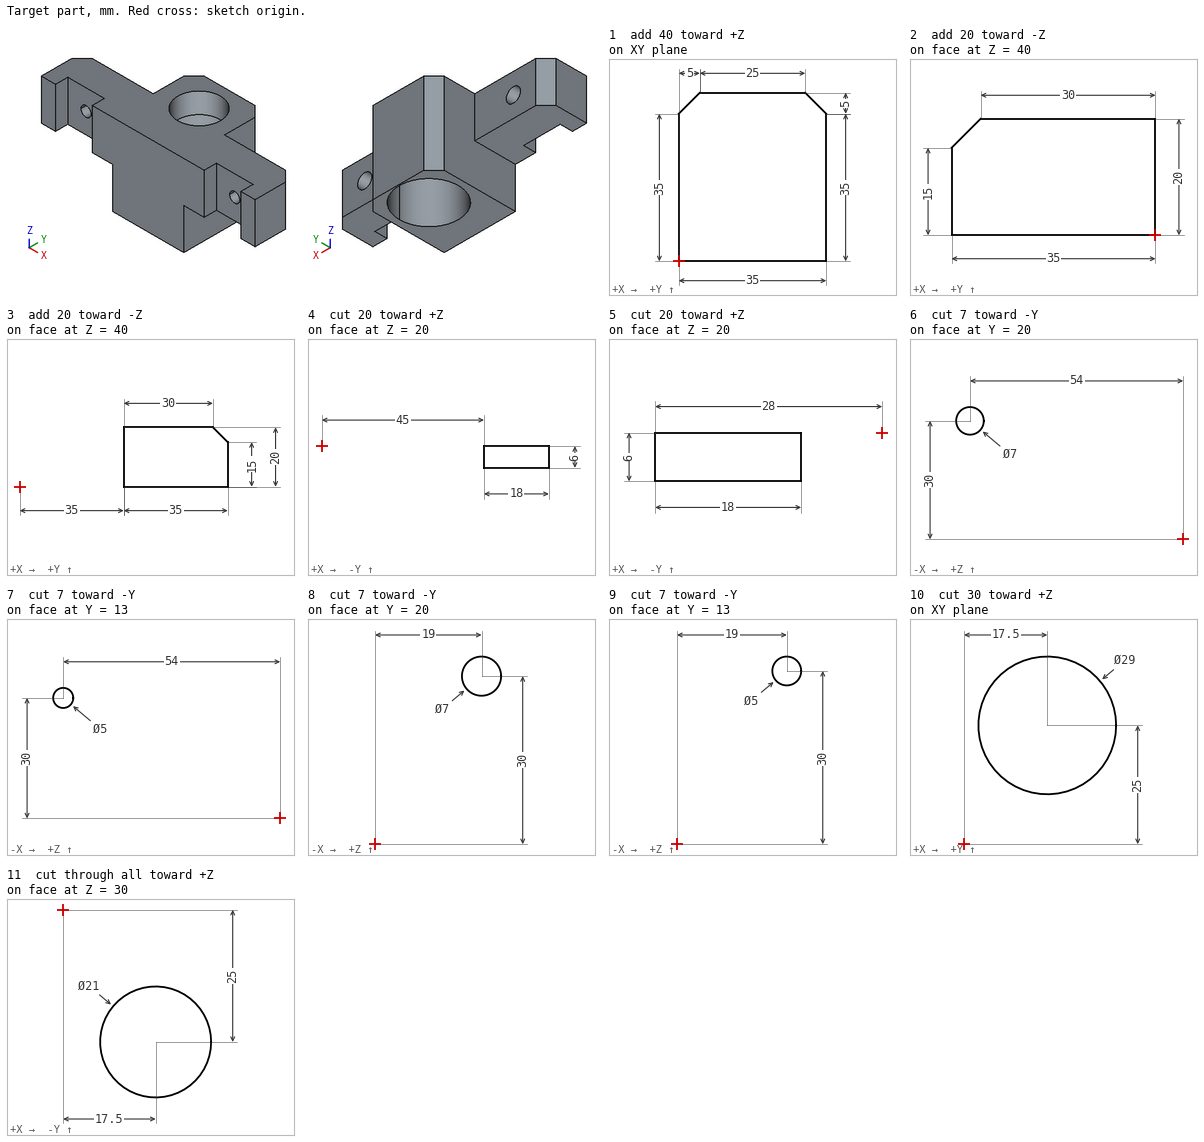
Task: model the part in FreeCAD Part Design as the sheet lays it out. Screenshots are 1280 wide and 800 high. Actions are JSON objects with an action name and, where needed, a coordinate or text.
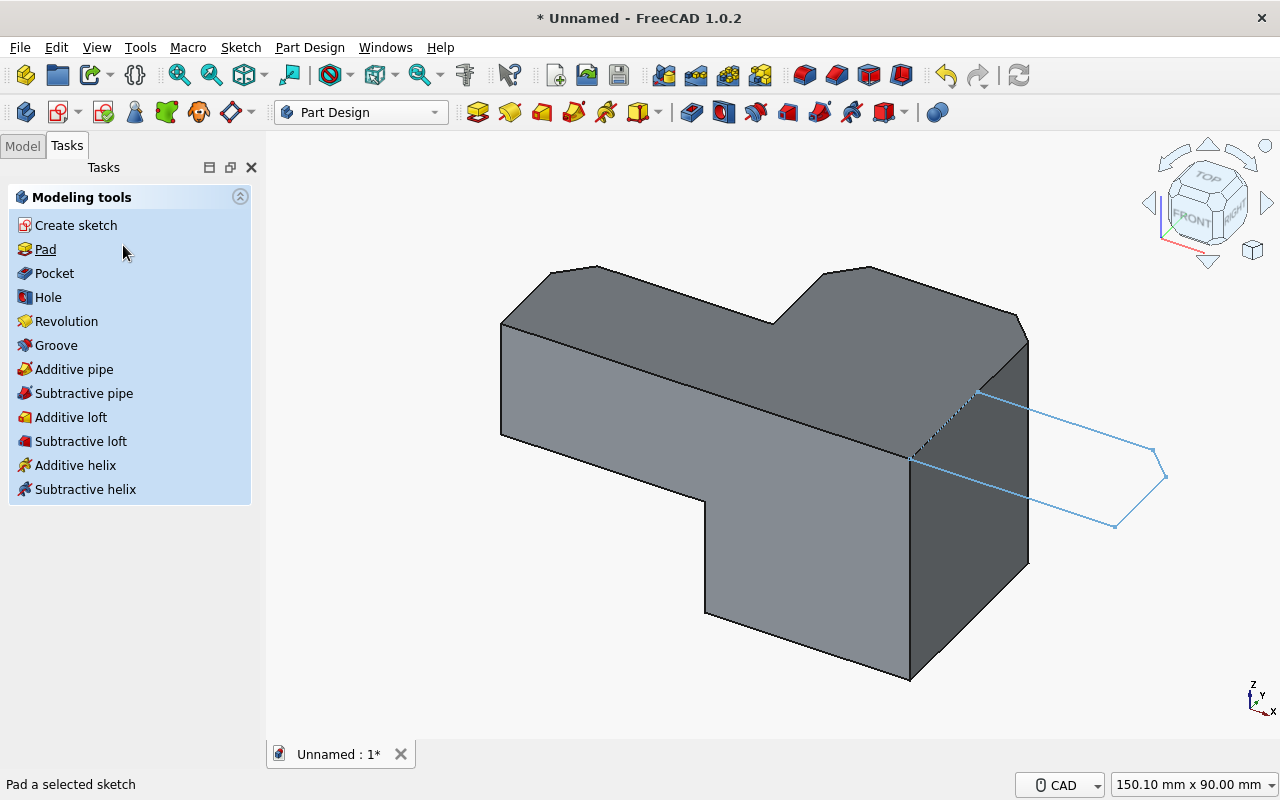
{"action": "left_click", "coordinate": [478, 112]}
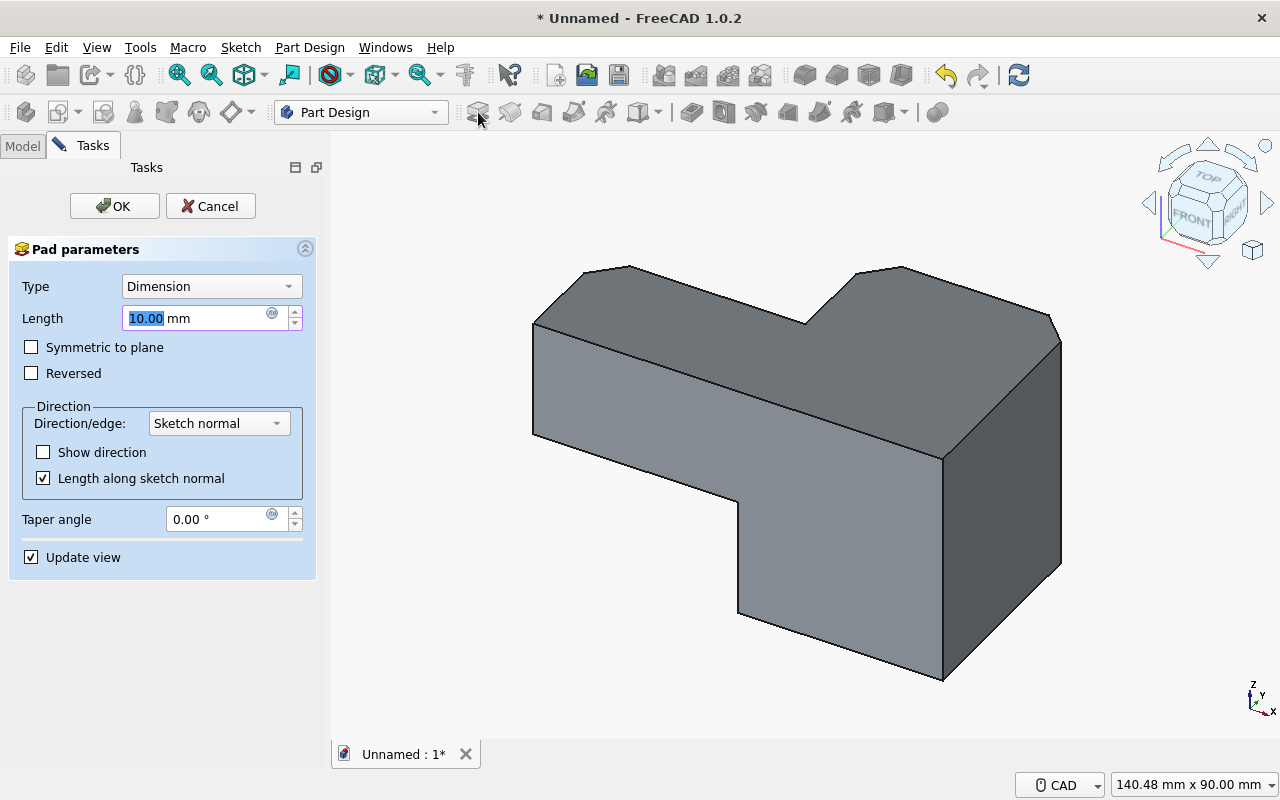
{"action": "type", "text": "20"}
{"action": "key", "text": "Tab"}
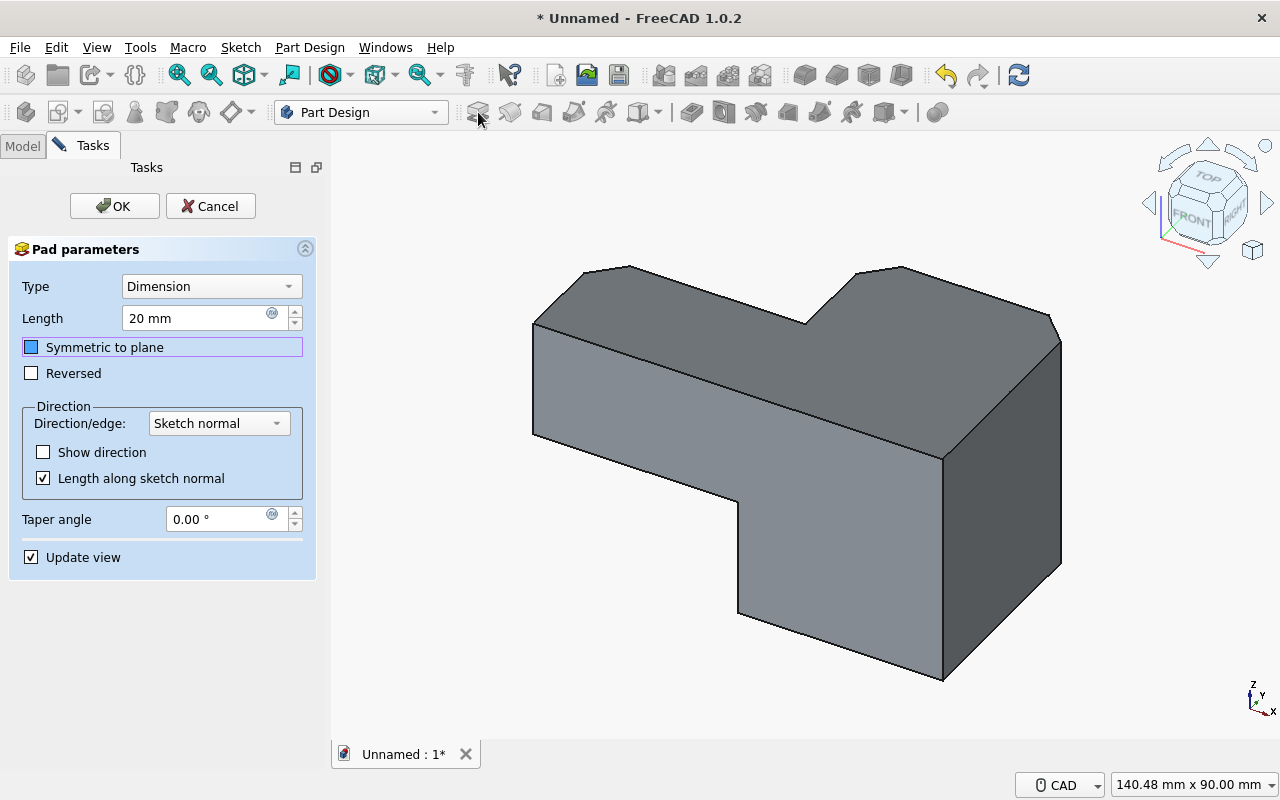
{"action": "left_click", "coordinate": [30, 373]}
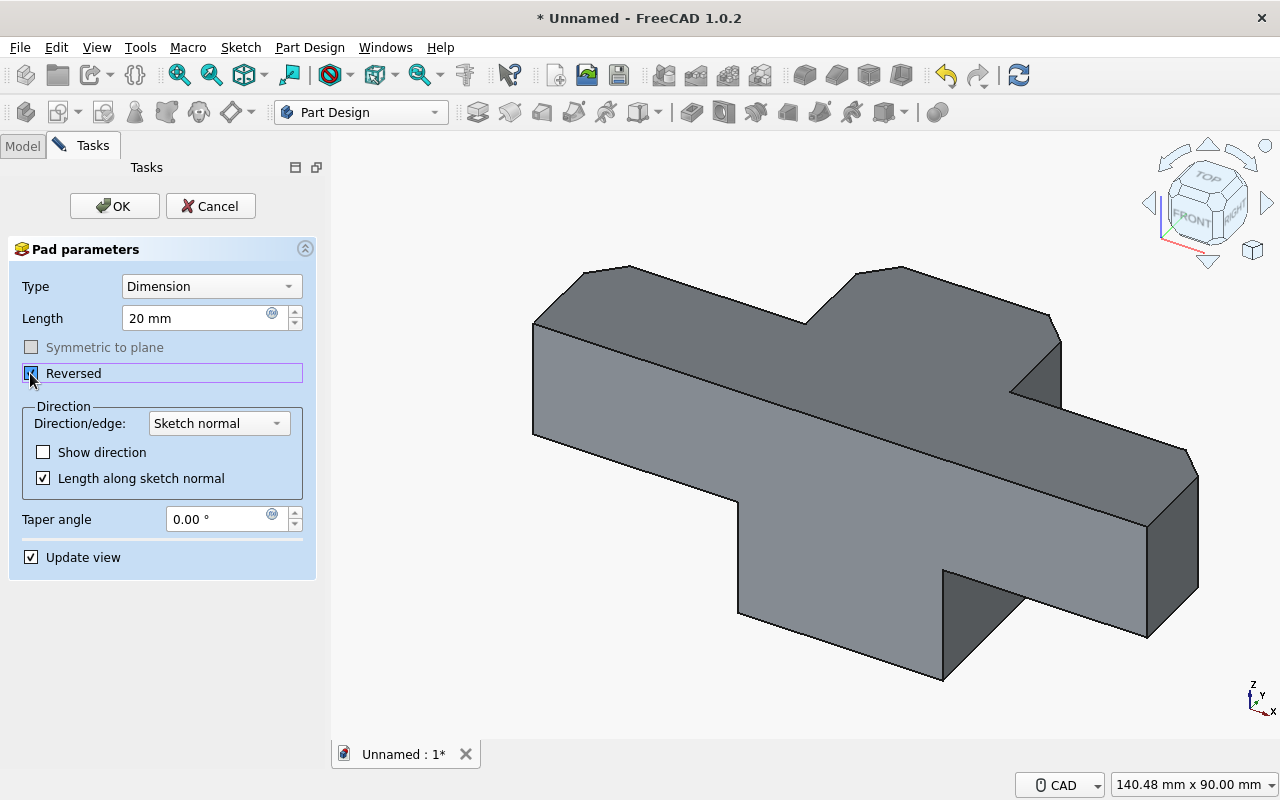
{"action": "left_click", "coordinate": [115, 206]}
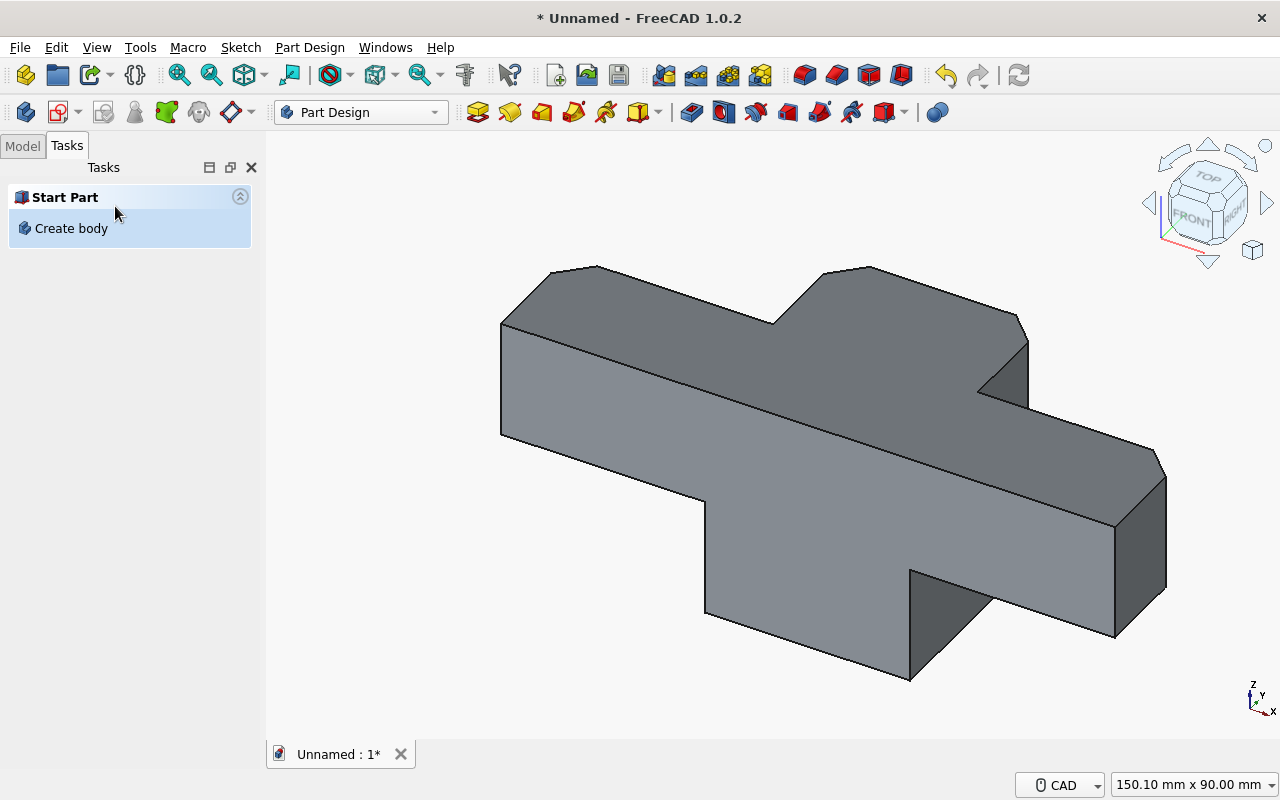
{"action": "left_click", "coordinate": [180, 76]}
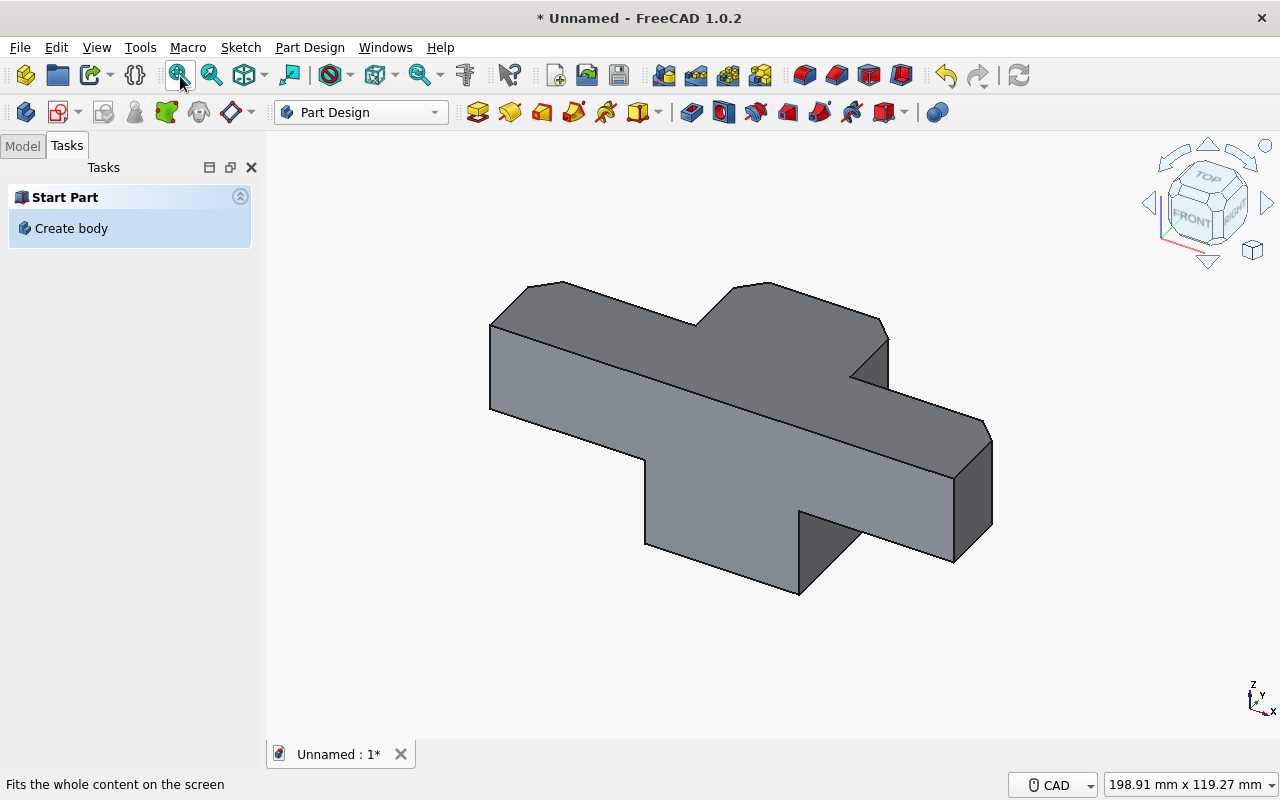
{"action": "key", "text": "5"}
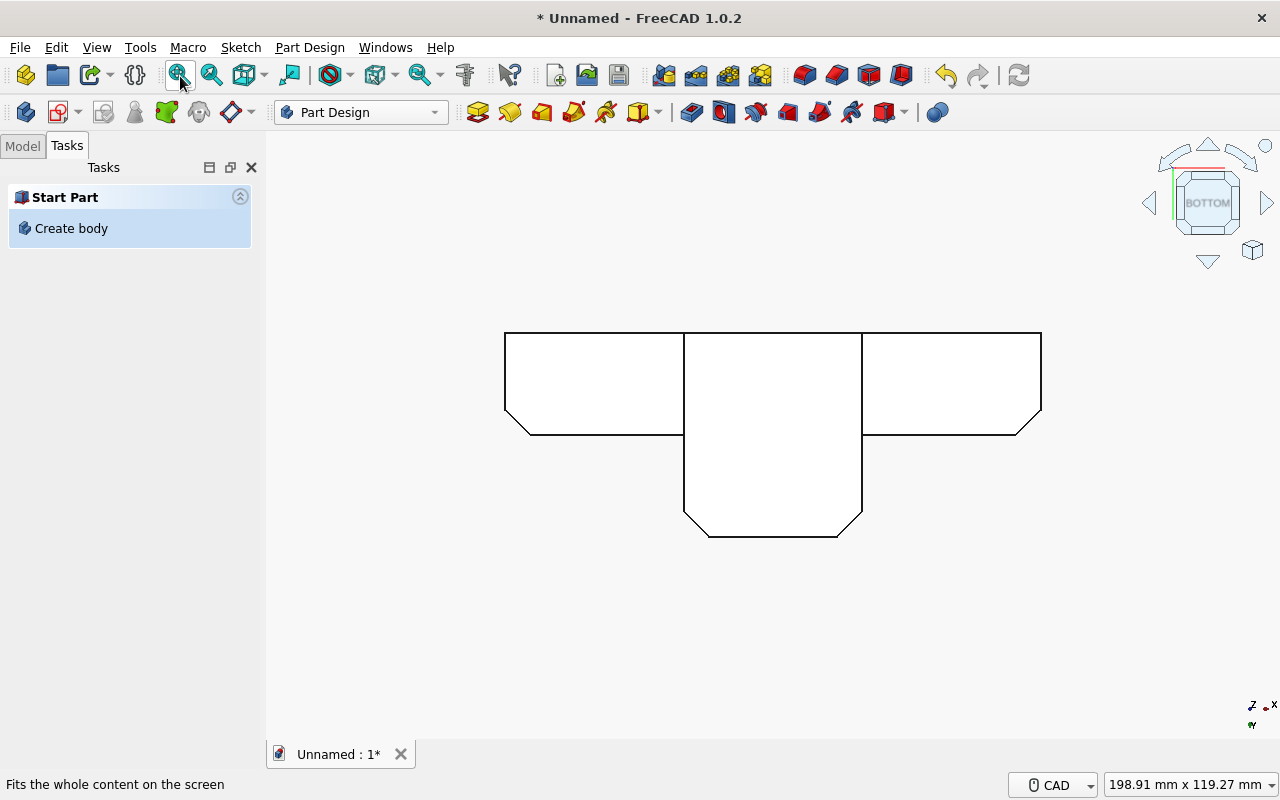
{"action": "left_click", "coordinate": [977, 383]}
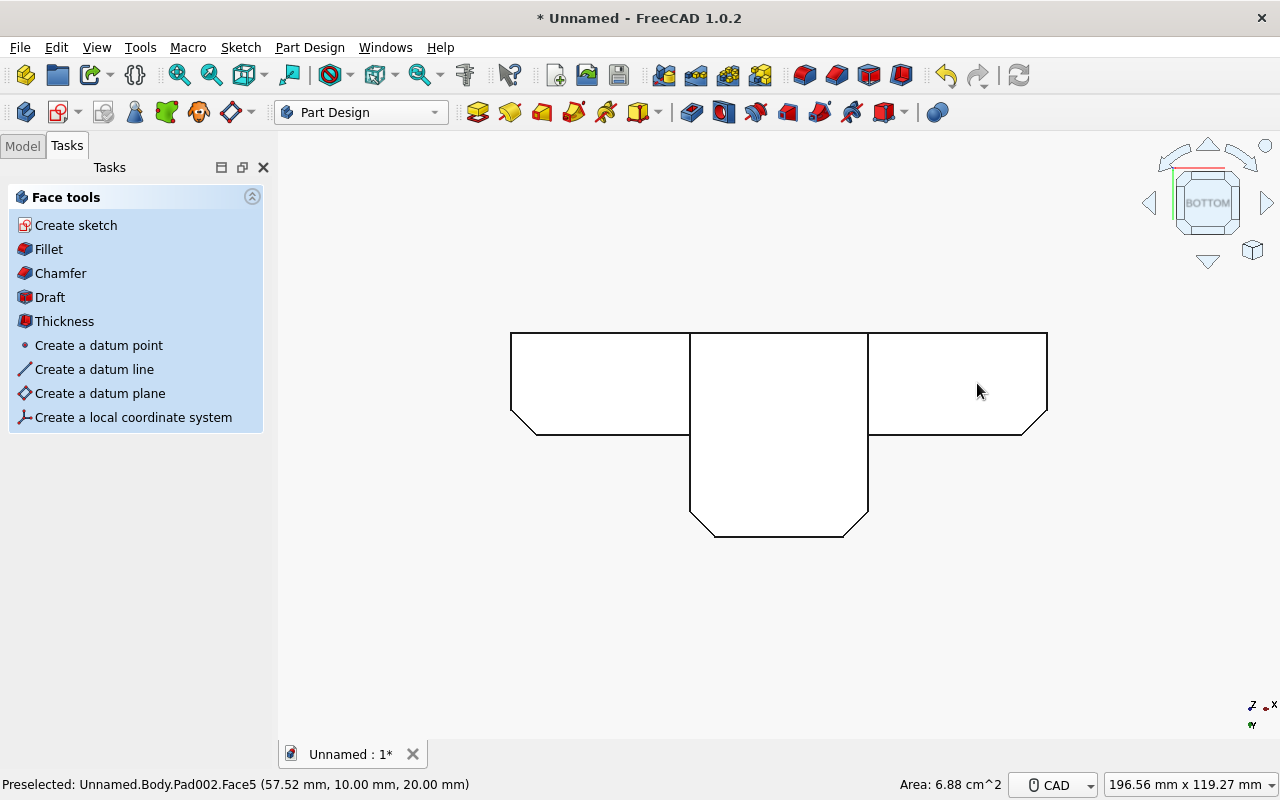
{"action": "left_click", "coordinate": [58, 112]}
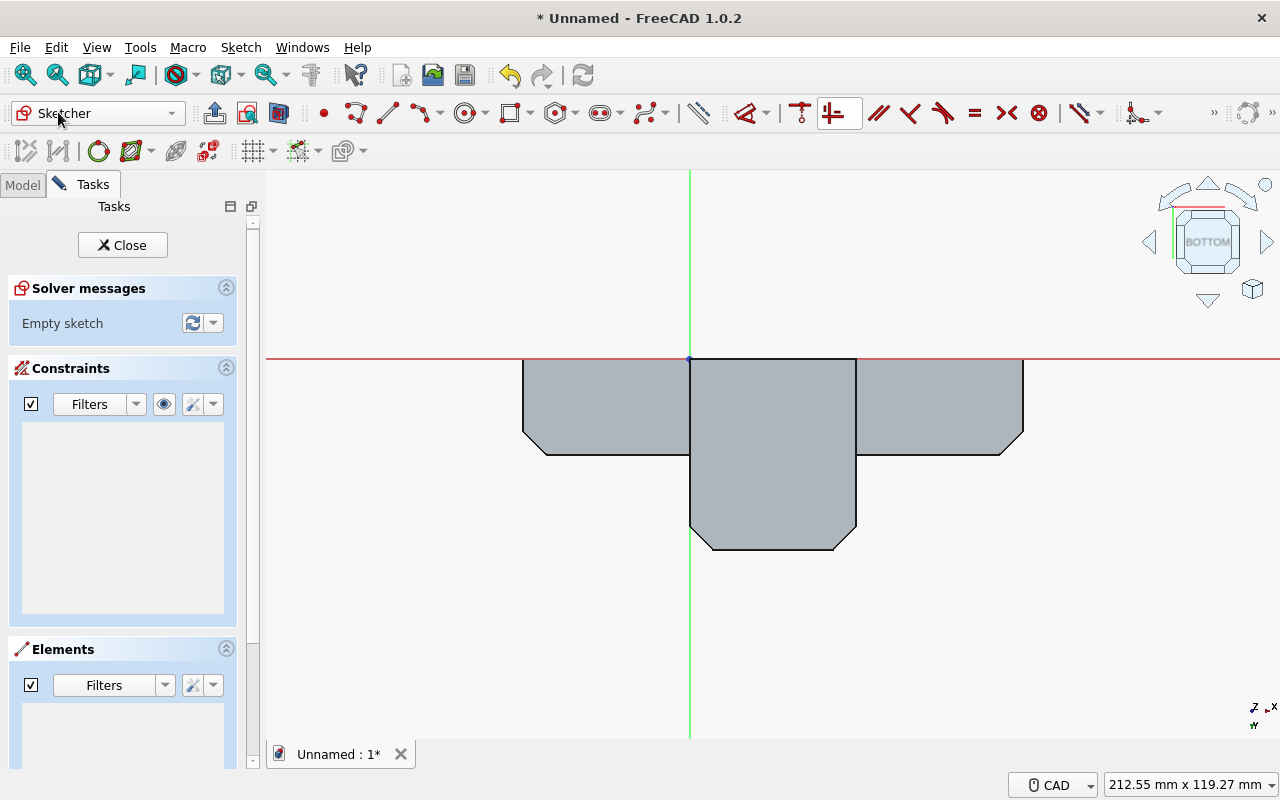
{"action": "scroll", "coordinate": [985, 361], "scroll_direction": "up", "scroll_amount": 10}